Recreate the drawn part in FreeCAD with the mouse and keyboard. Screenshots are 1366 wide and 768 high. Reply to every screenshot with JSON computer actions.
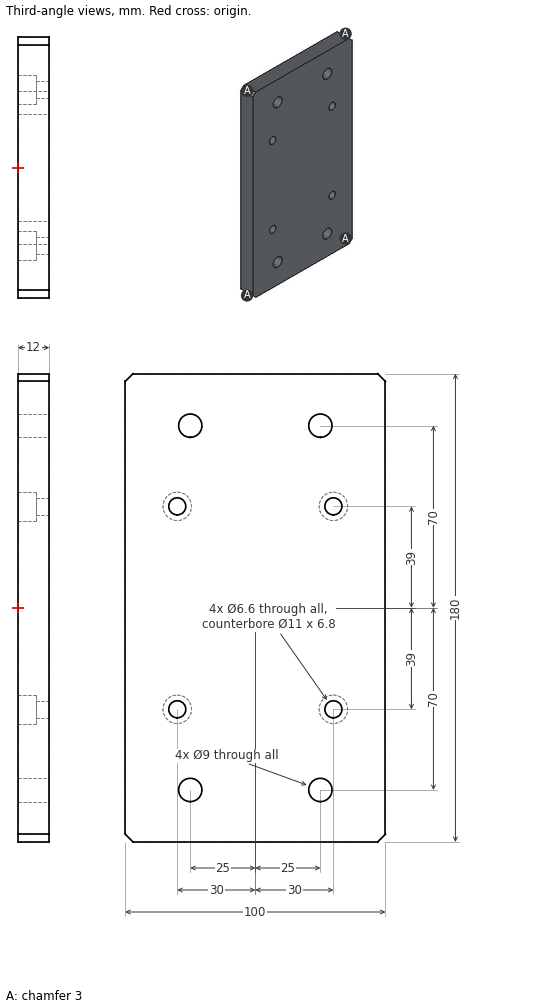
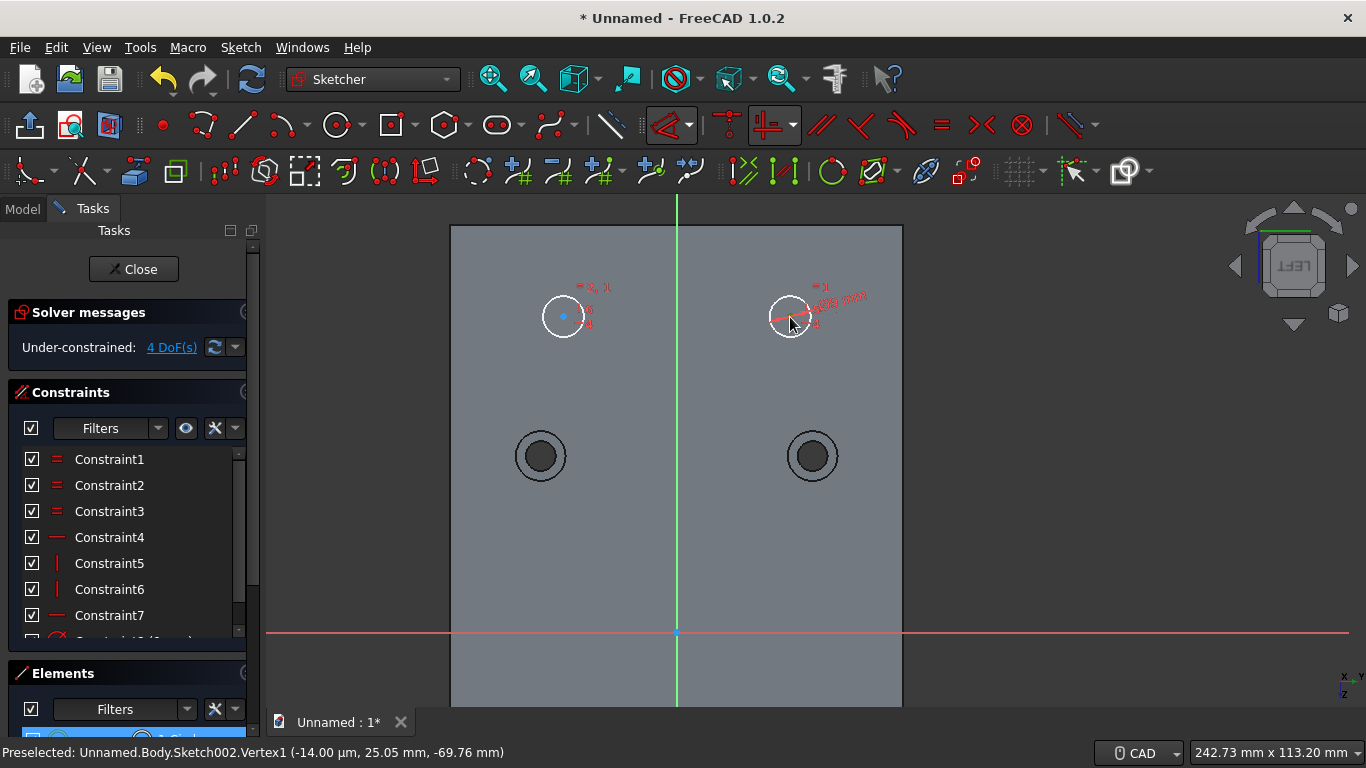
{"action": "left_click", "coordinate": [692, 126]}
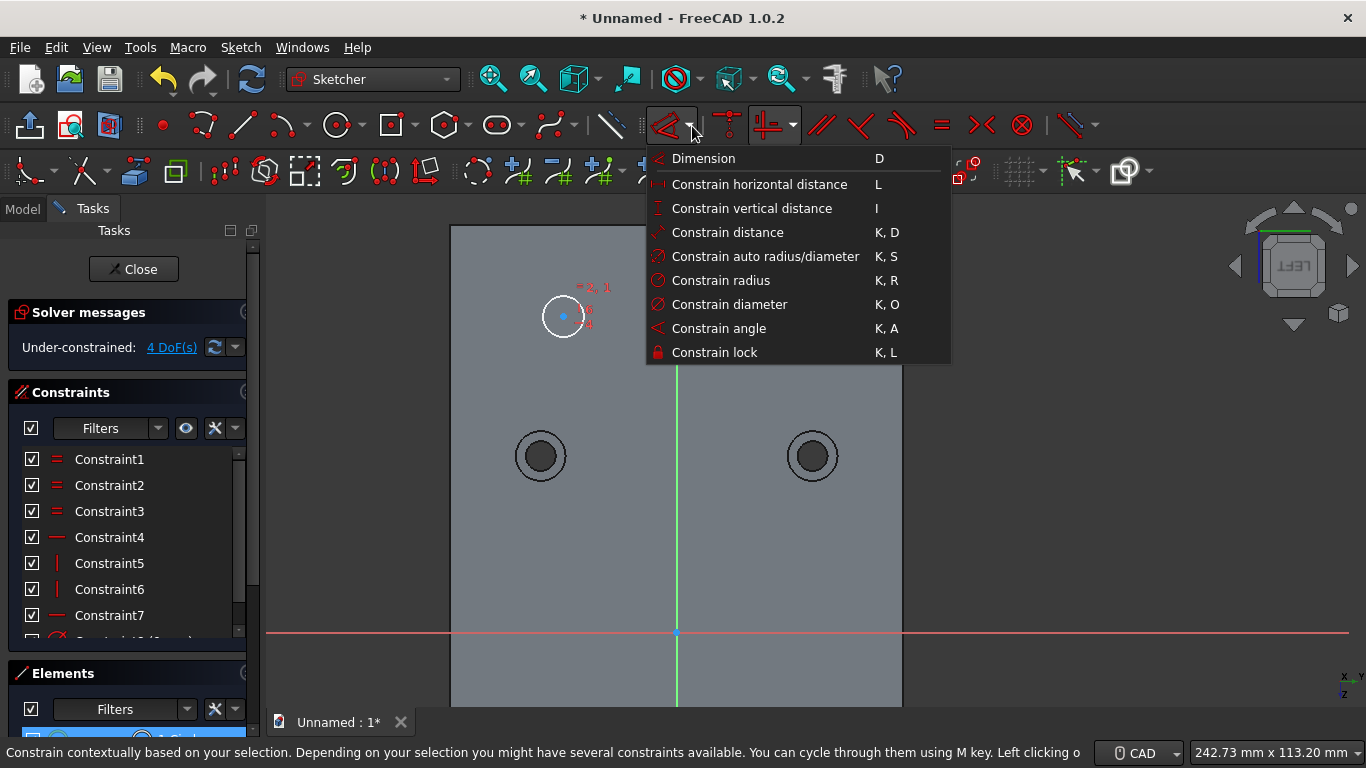
{"action": "left_click", "coordinate": [799, 184]}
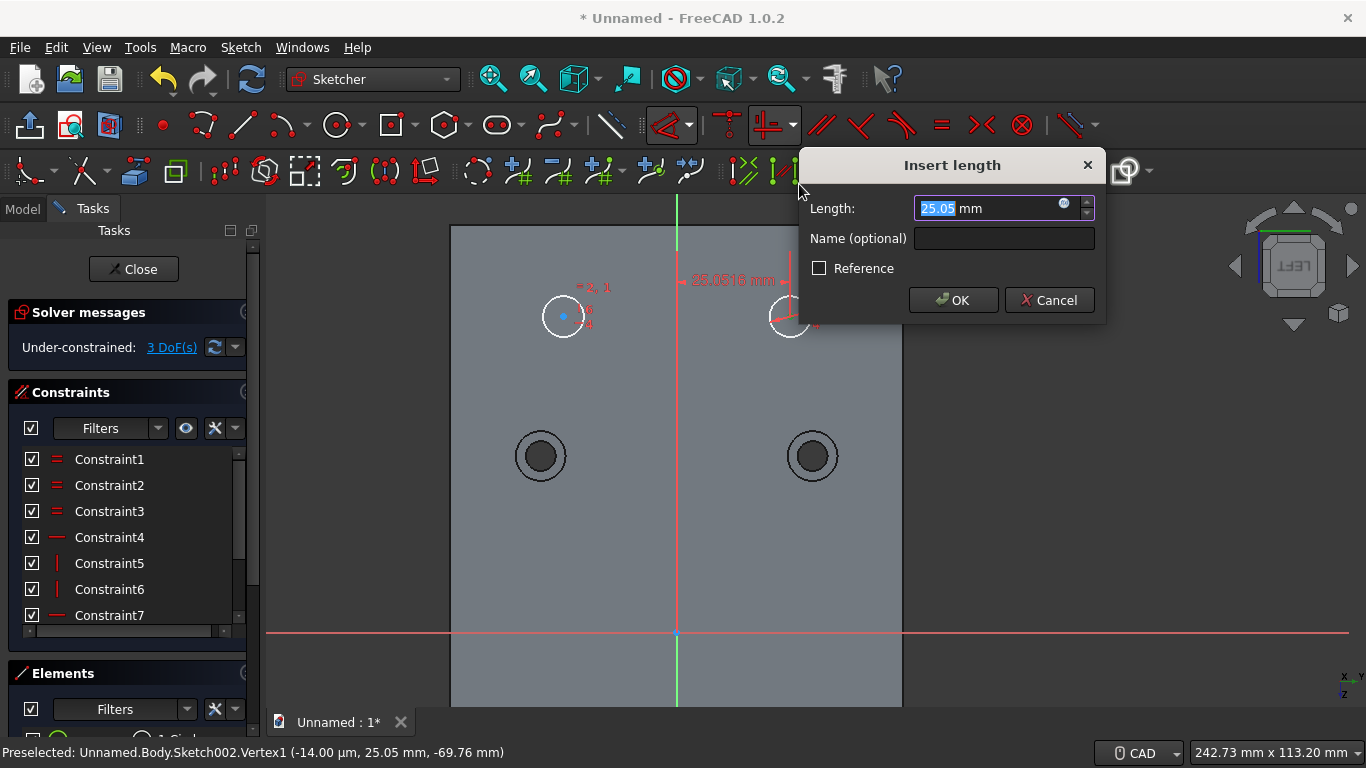
{"action": "type", "text": "25"}
{"action": "key", "text": "Return"}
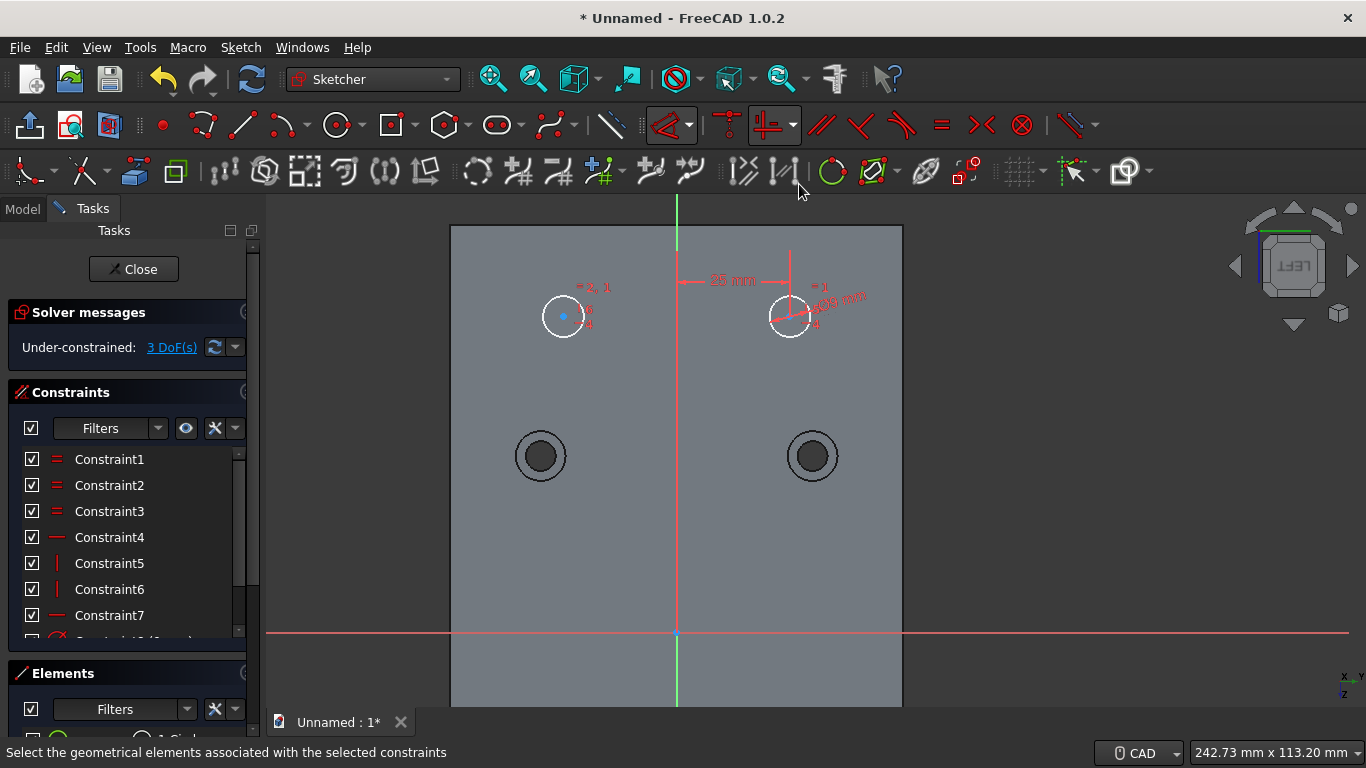
{"action": "left_click", "coordinate": [790, 317]}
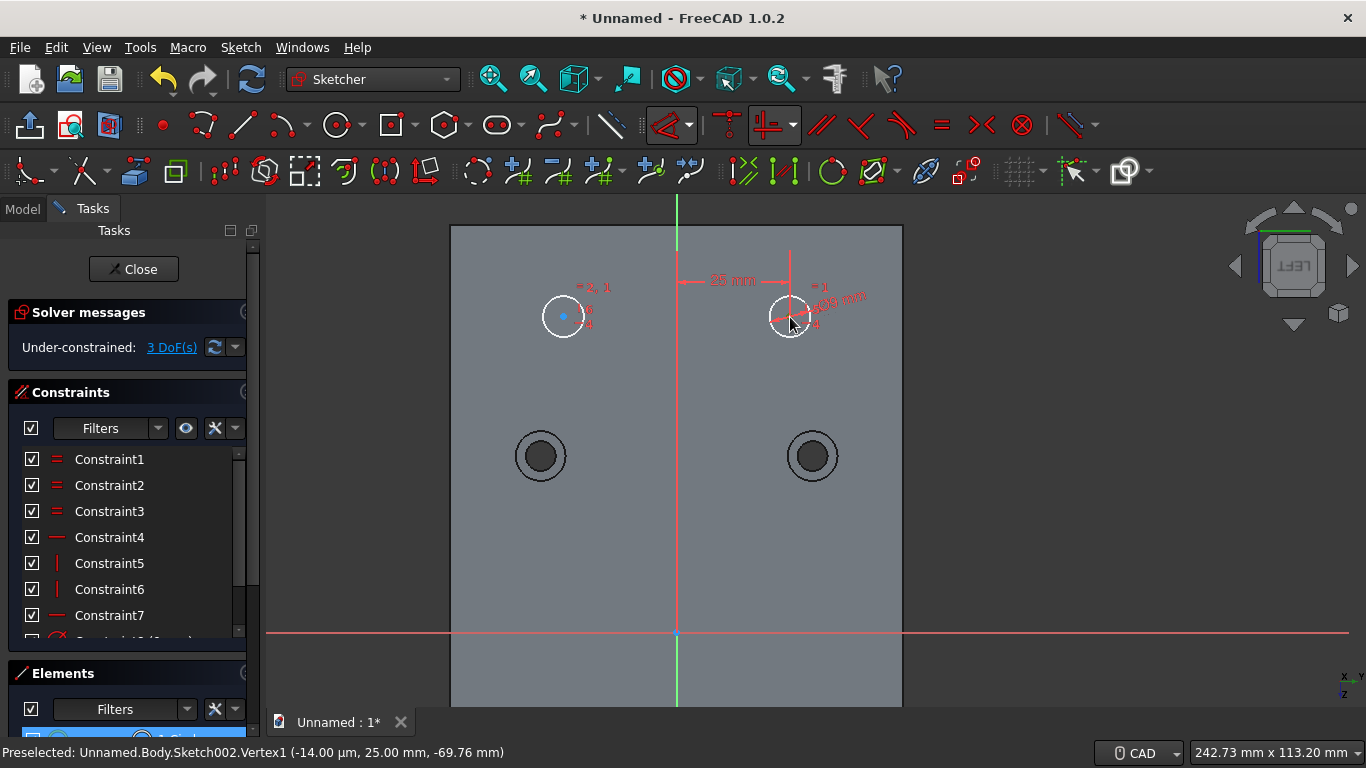
{"action": "key", "text": "i"}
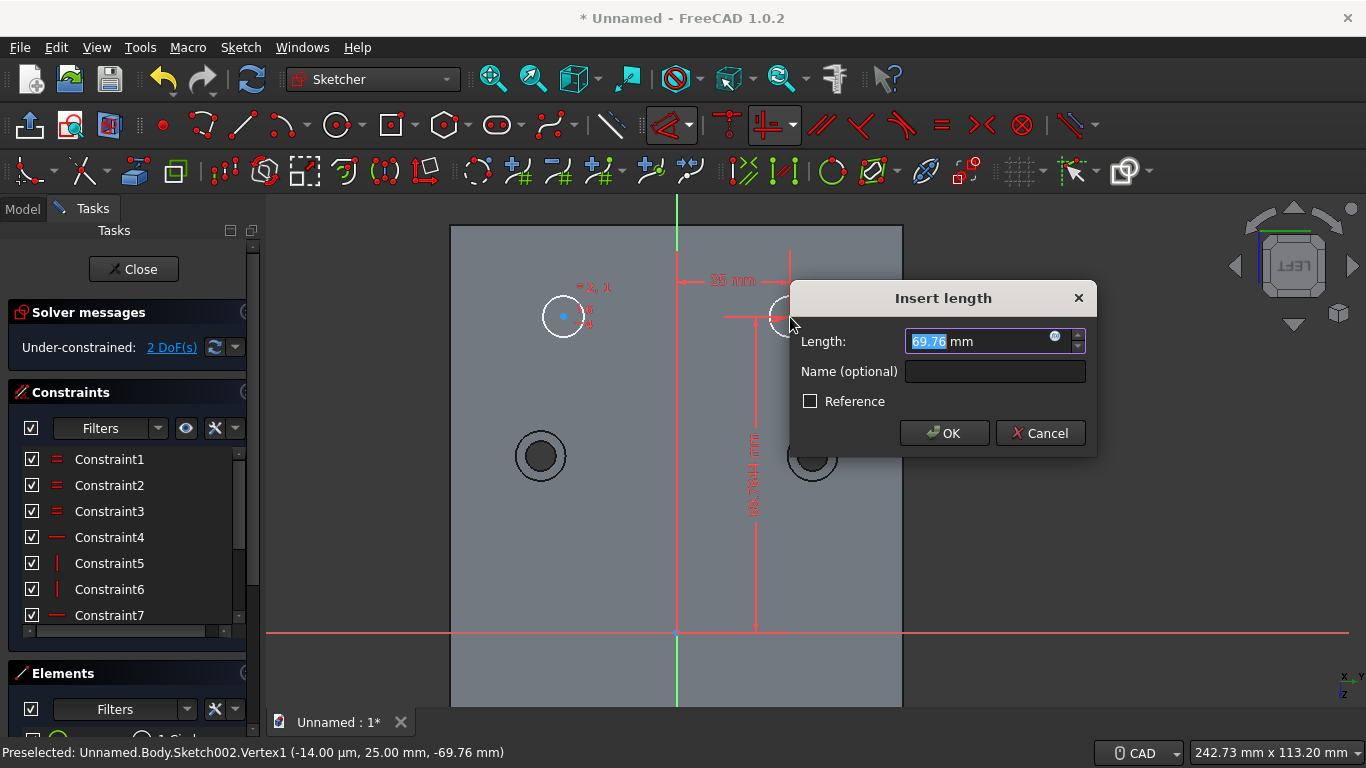
{"action": "type", "text": "70"}
{"action": "key", "text": "Return"}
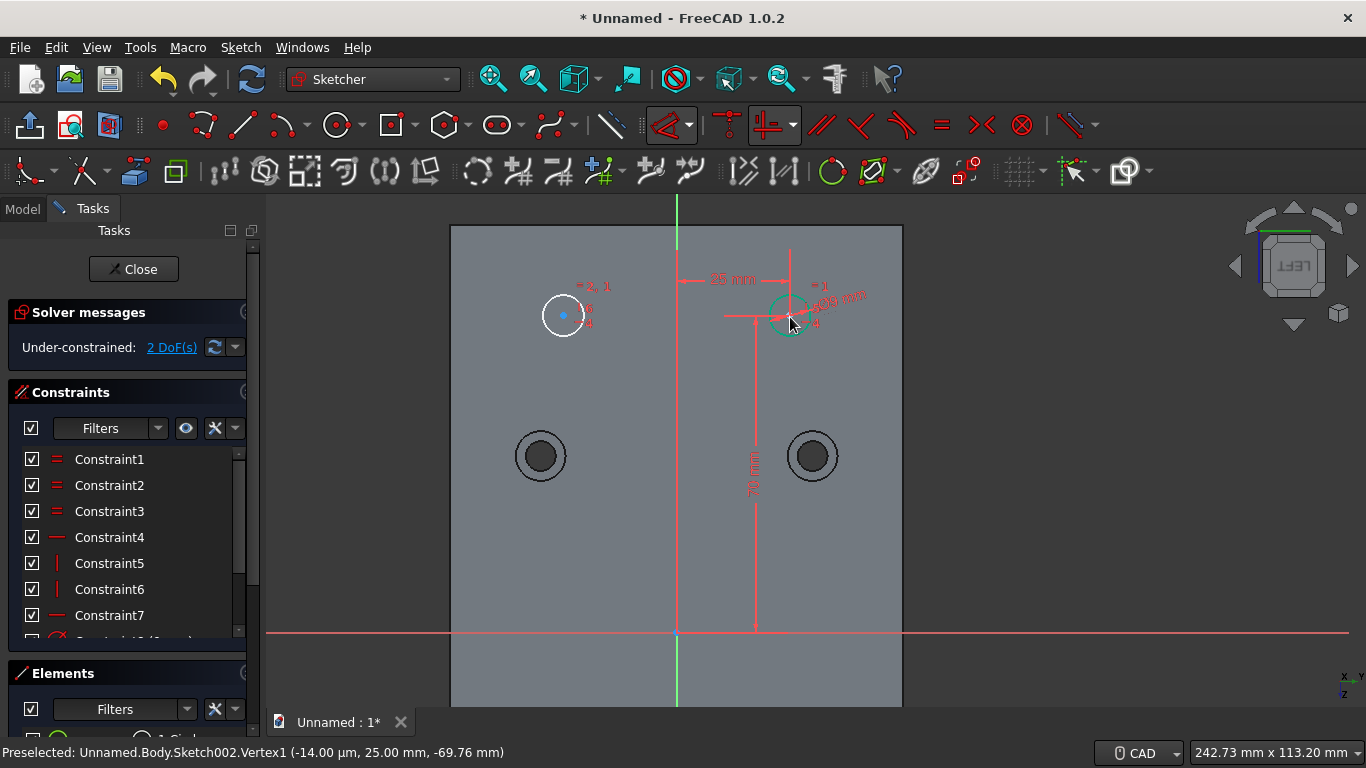
{"action": "left_click", "coordinate": [563, 316]}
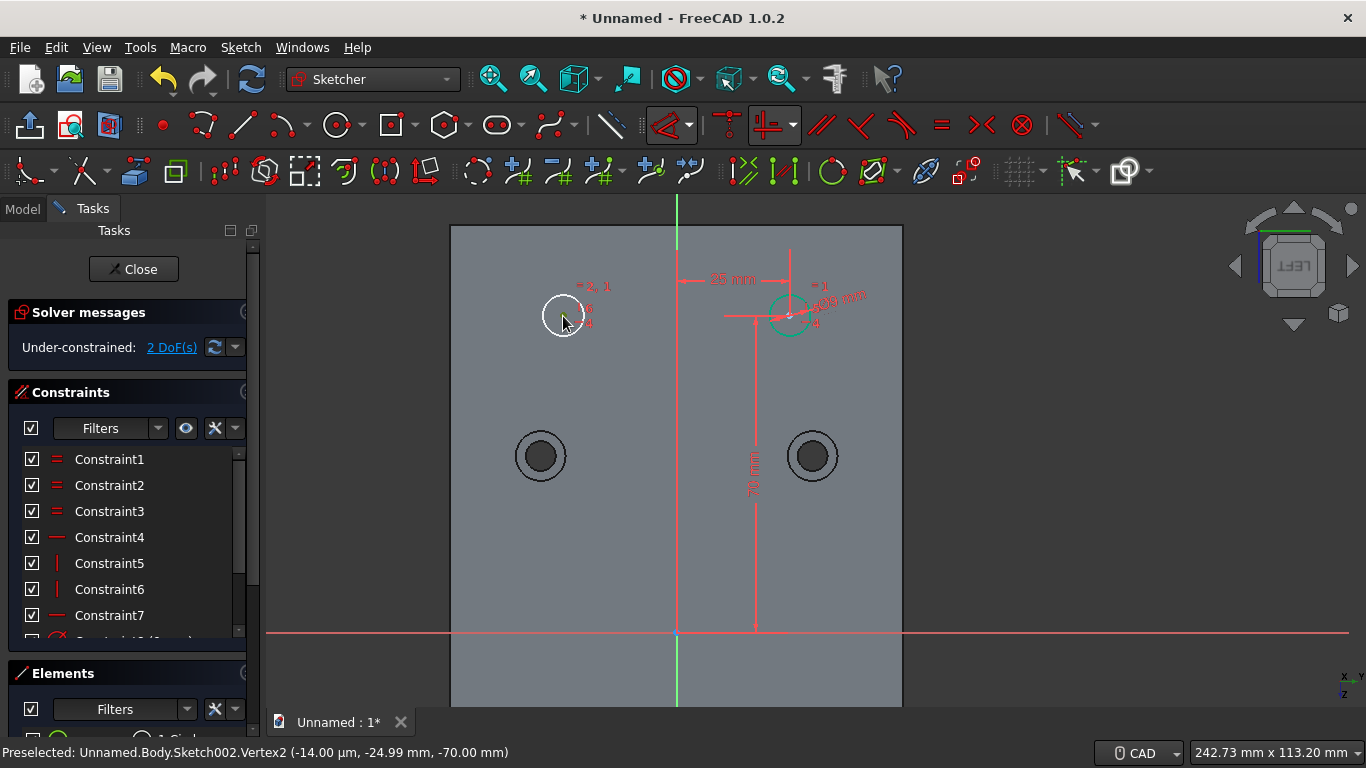
{"action": "key", "text": "l"}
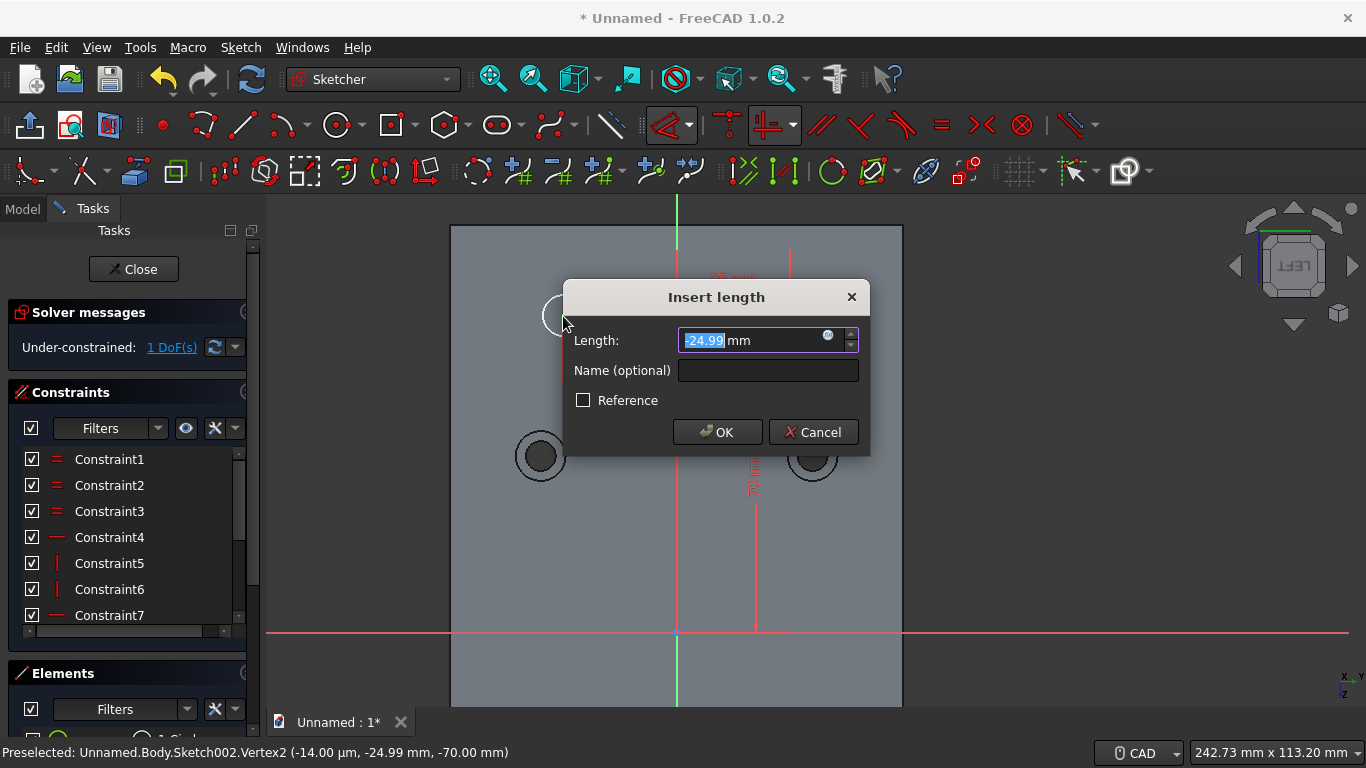
{"action": "type", "text": "-25"}
{"action": "key", "text": "Return"}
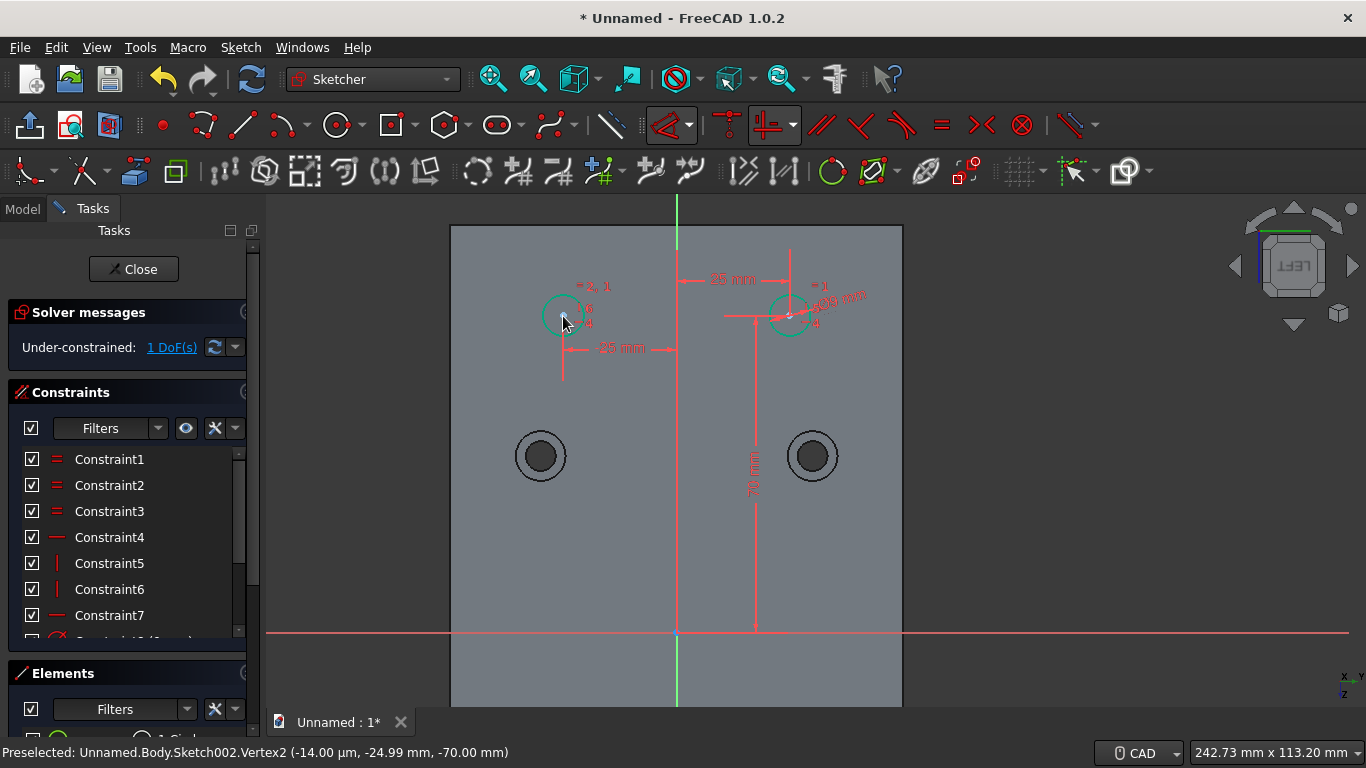
{"action": "scroll", "coordinate": [805, 302], "scroll_direction": "down", "scroll_amount": 4}